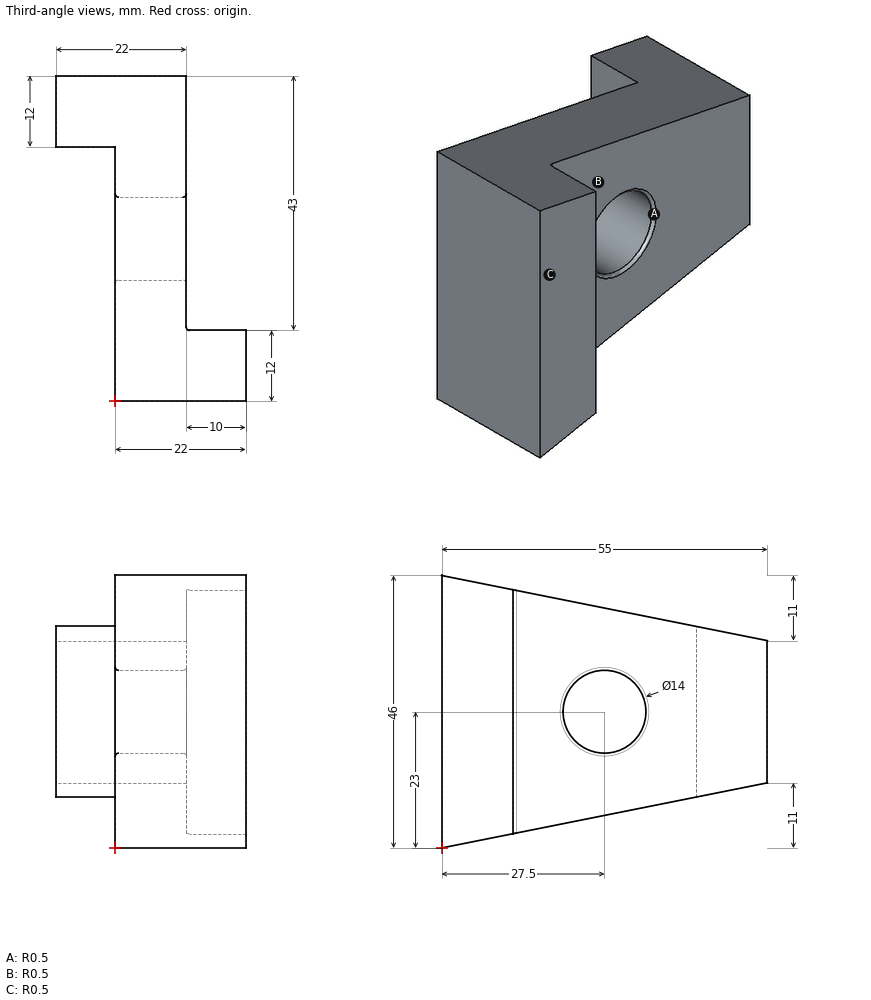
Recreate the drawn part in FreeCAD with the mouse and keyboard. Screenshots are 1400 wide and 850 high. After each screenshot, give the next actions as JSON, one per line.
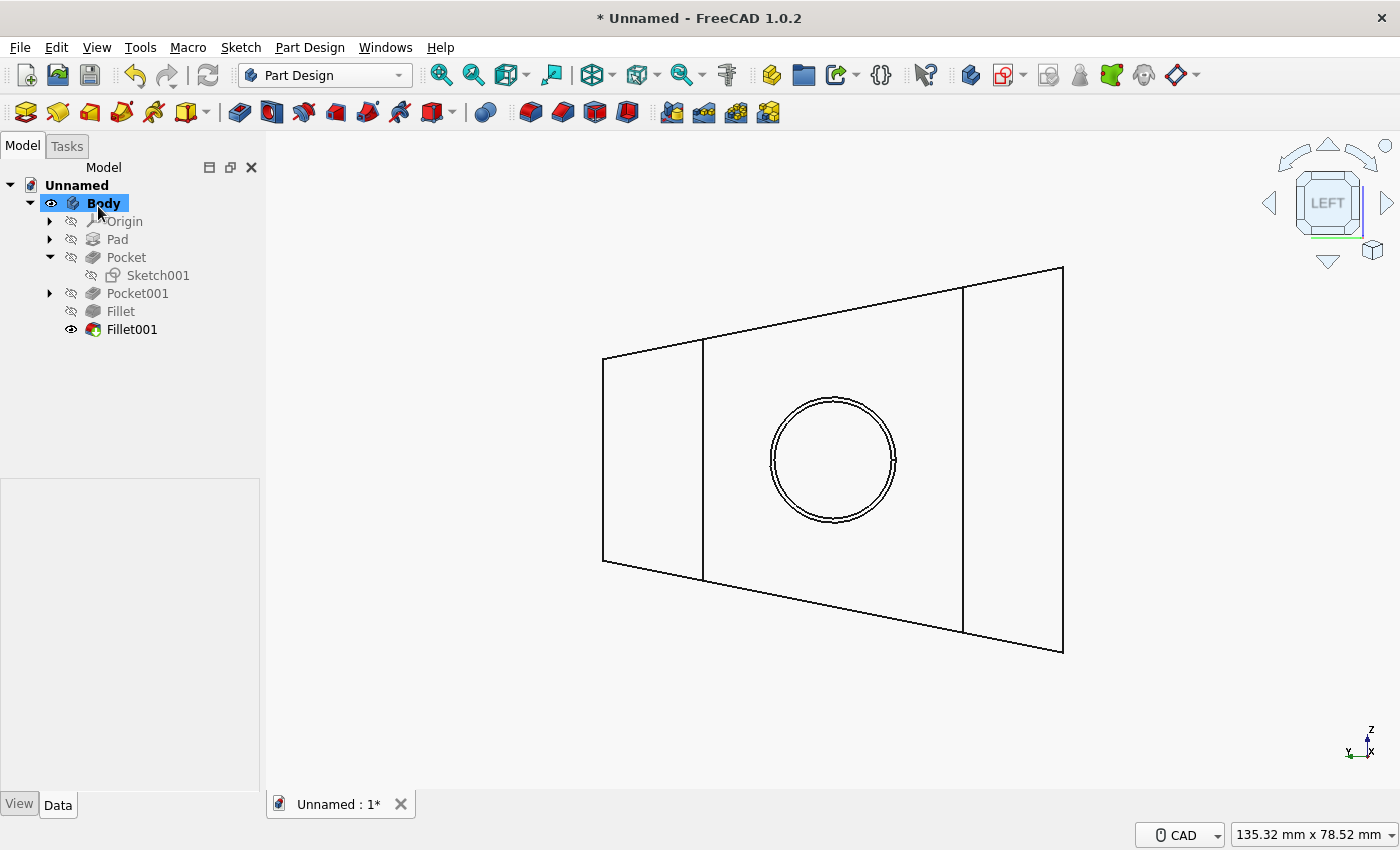
{"action": "key", "text": "0"}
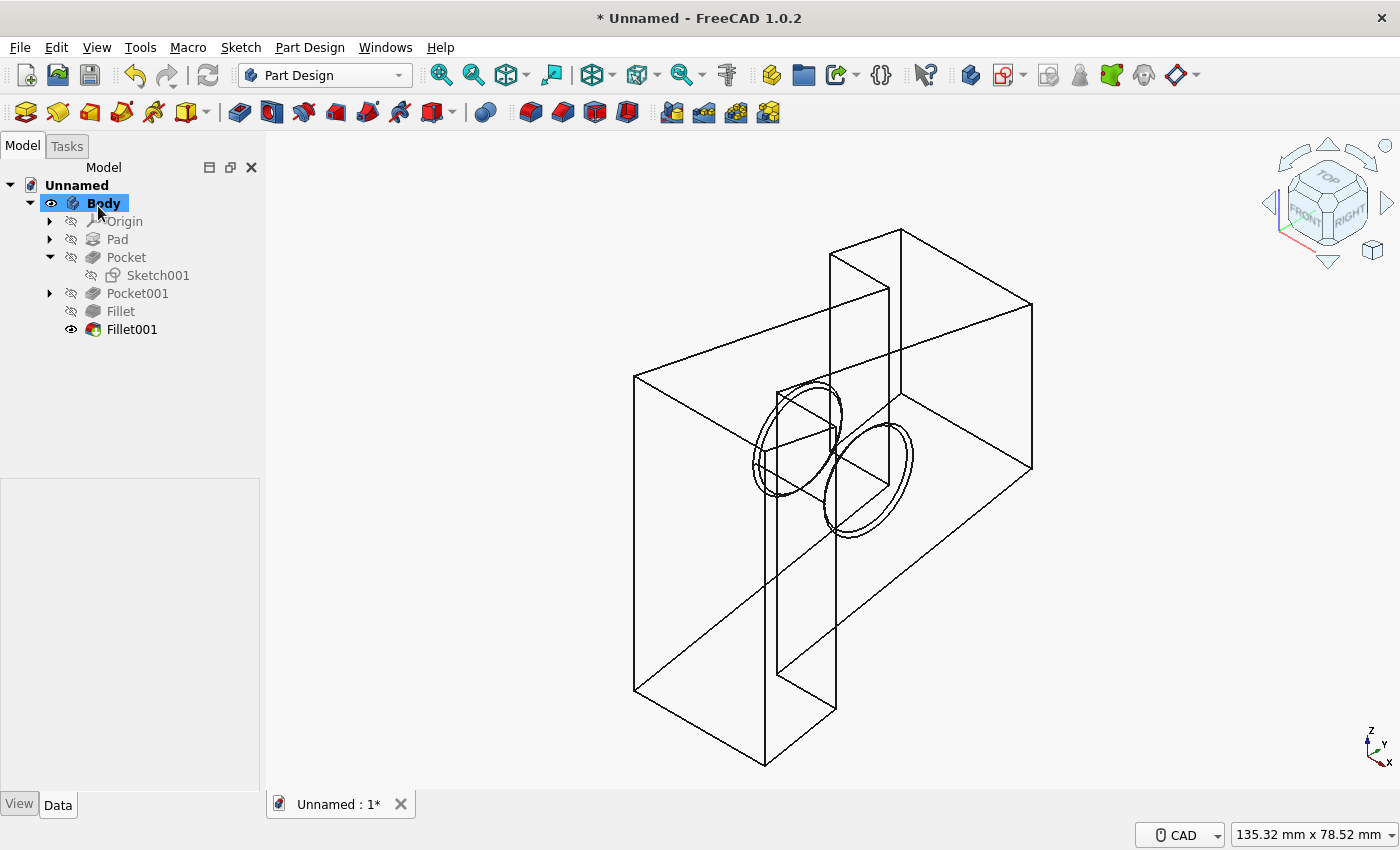
{"action": "left_click", "coordinate": [777, 533]}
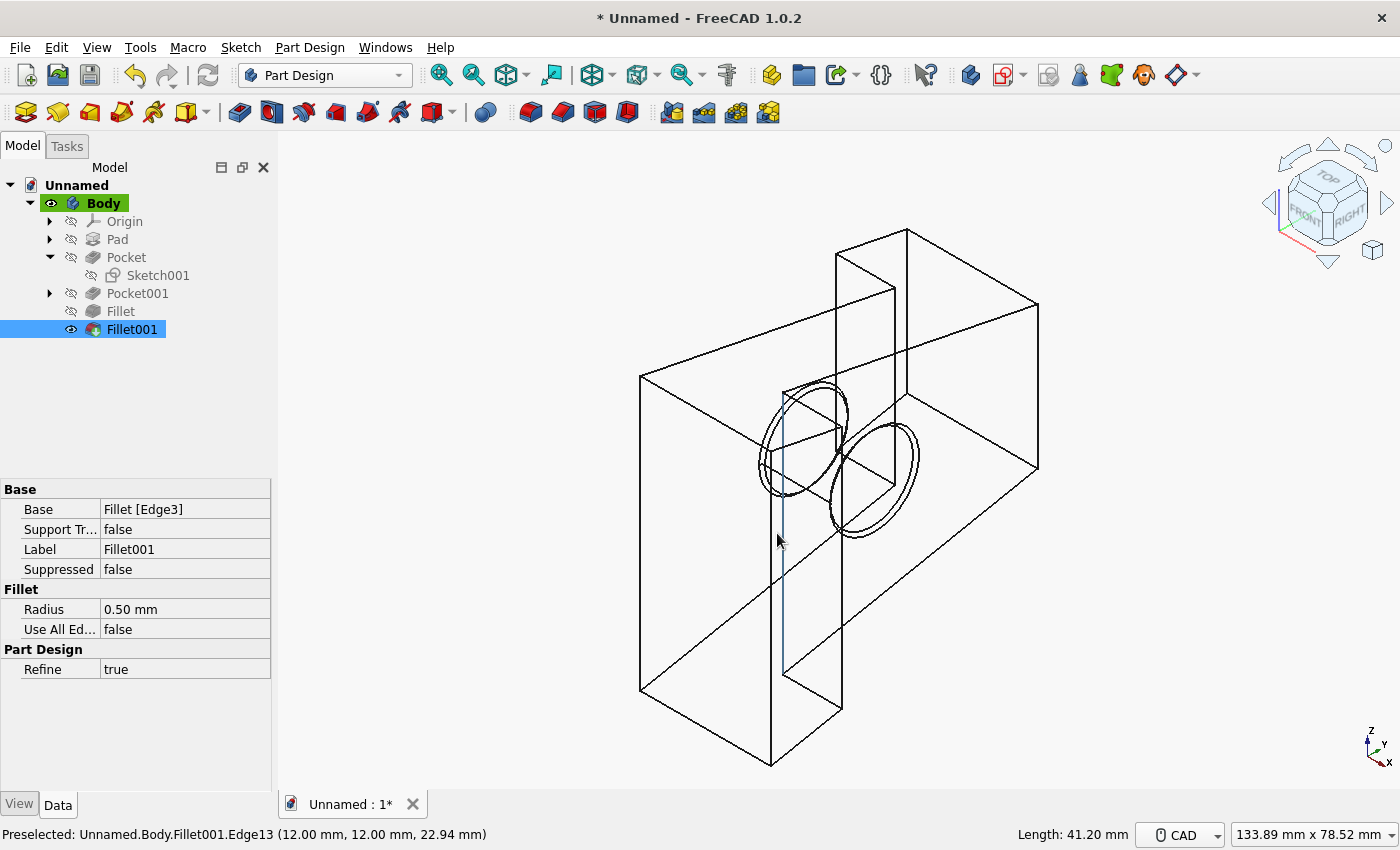
{"action": "key", "text": "v 1"}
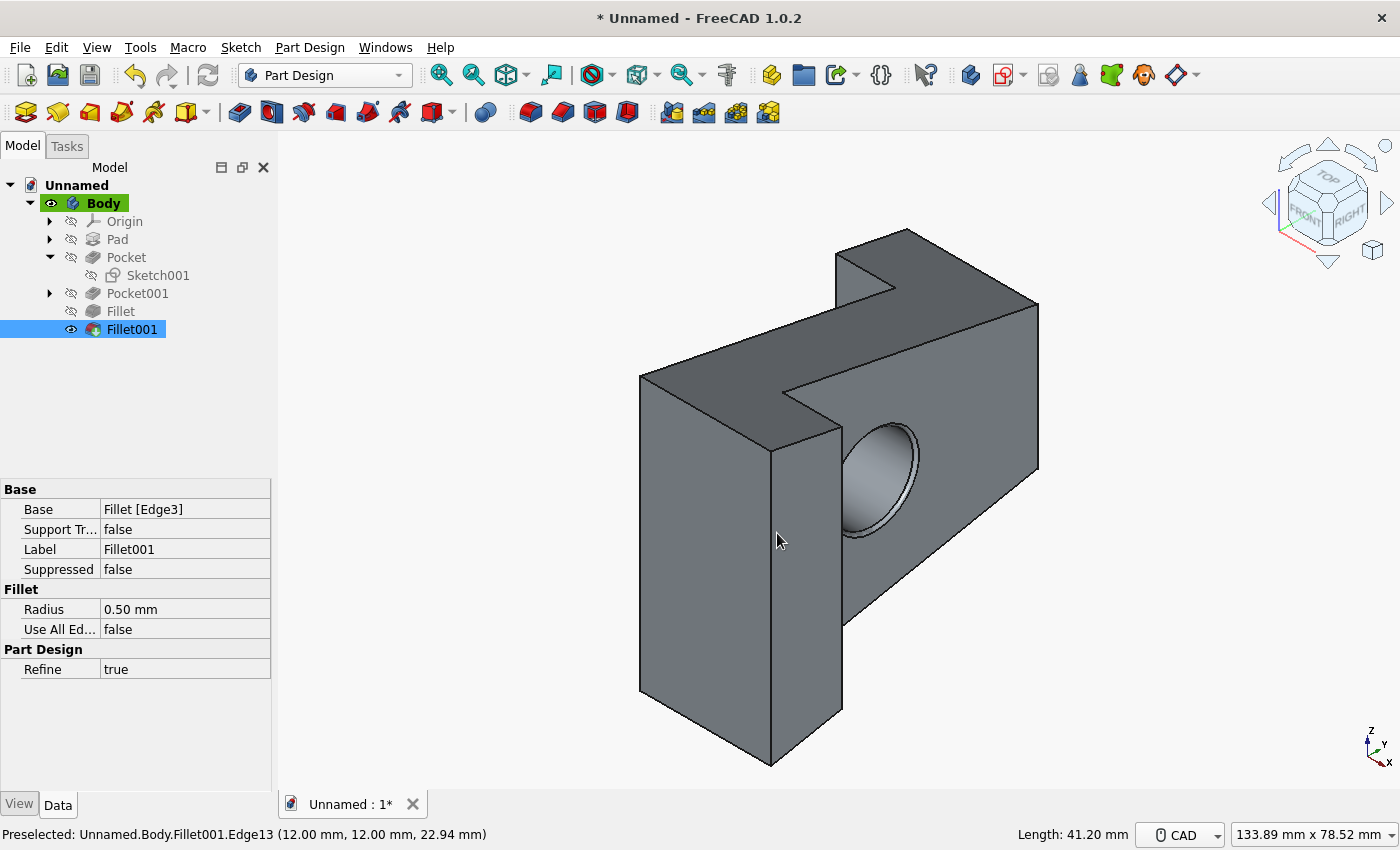
{"action": "left_click", "coordinate": [532, 112]}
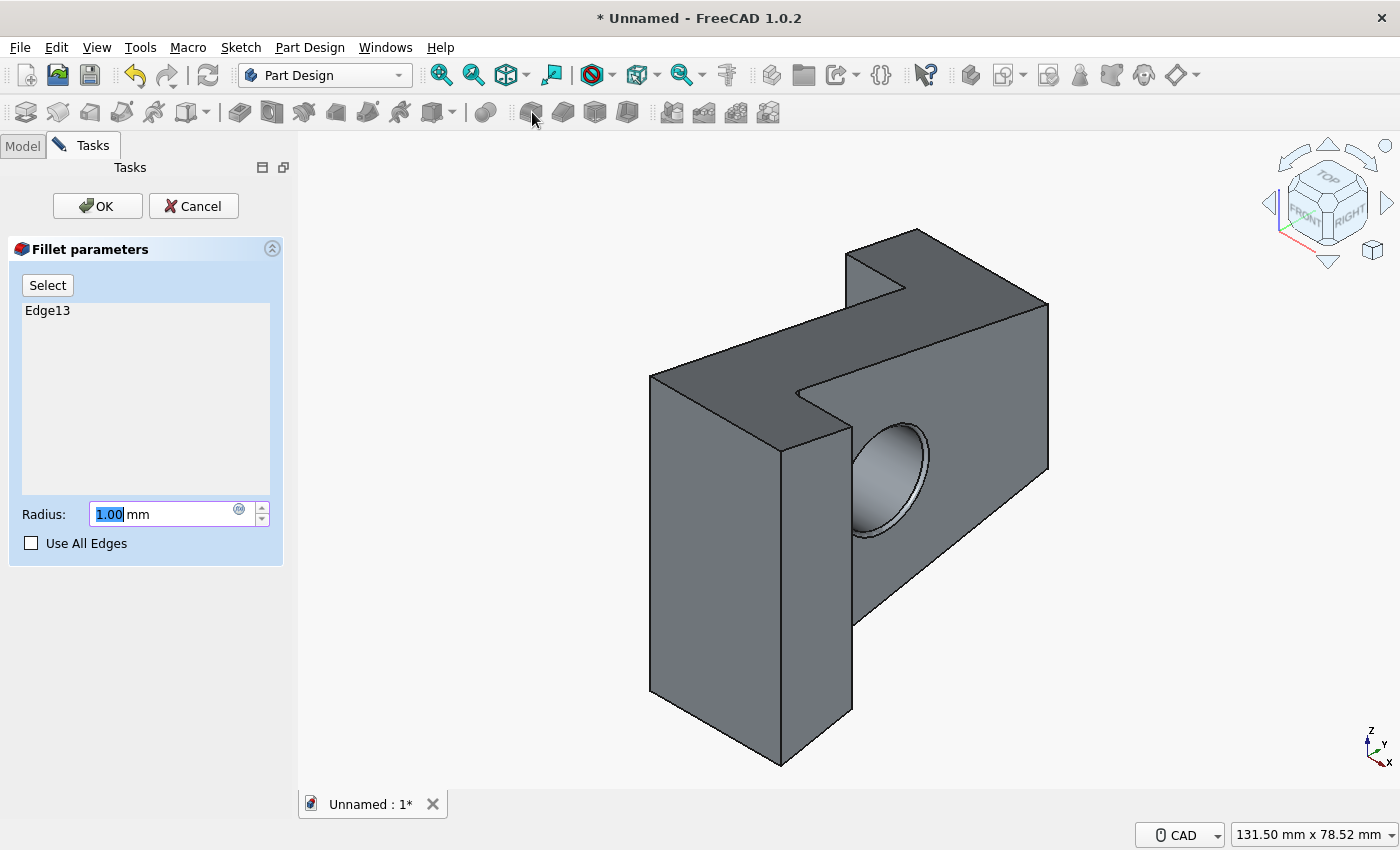
{"action": "type", "text": "0.5"}
{"action": "key", "text": "Tab"}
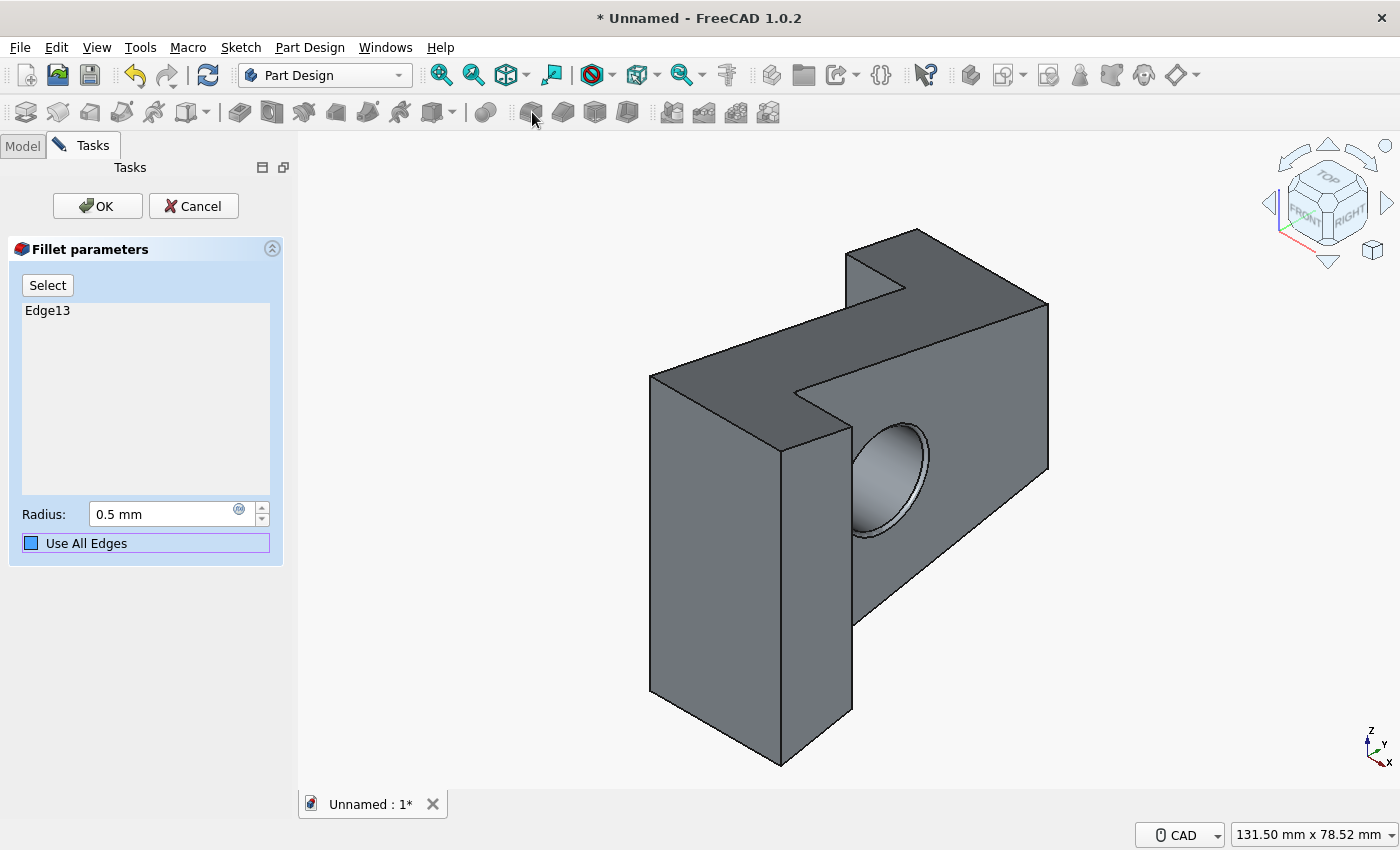
{"action": "left_click", "coordinate": [98, 206]}